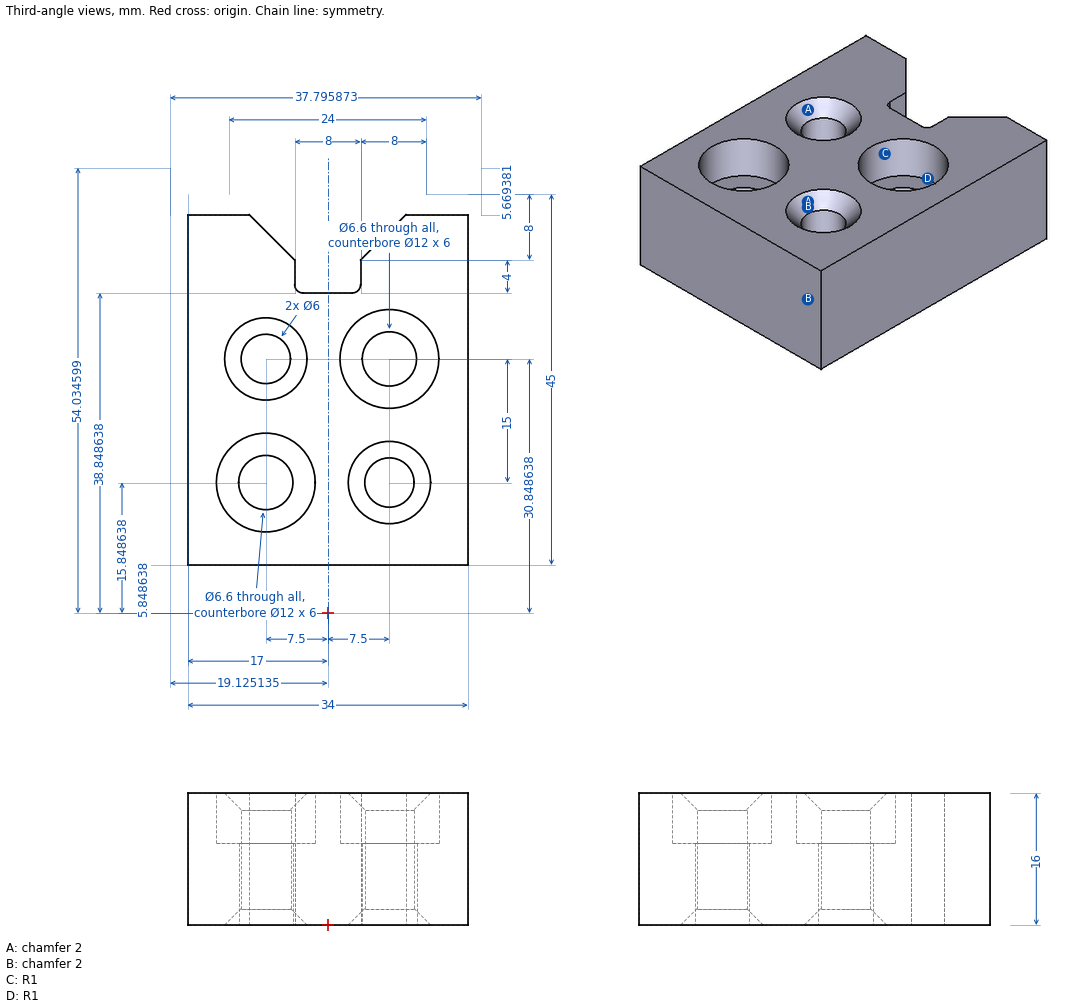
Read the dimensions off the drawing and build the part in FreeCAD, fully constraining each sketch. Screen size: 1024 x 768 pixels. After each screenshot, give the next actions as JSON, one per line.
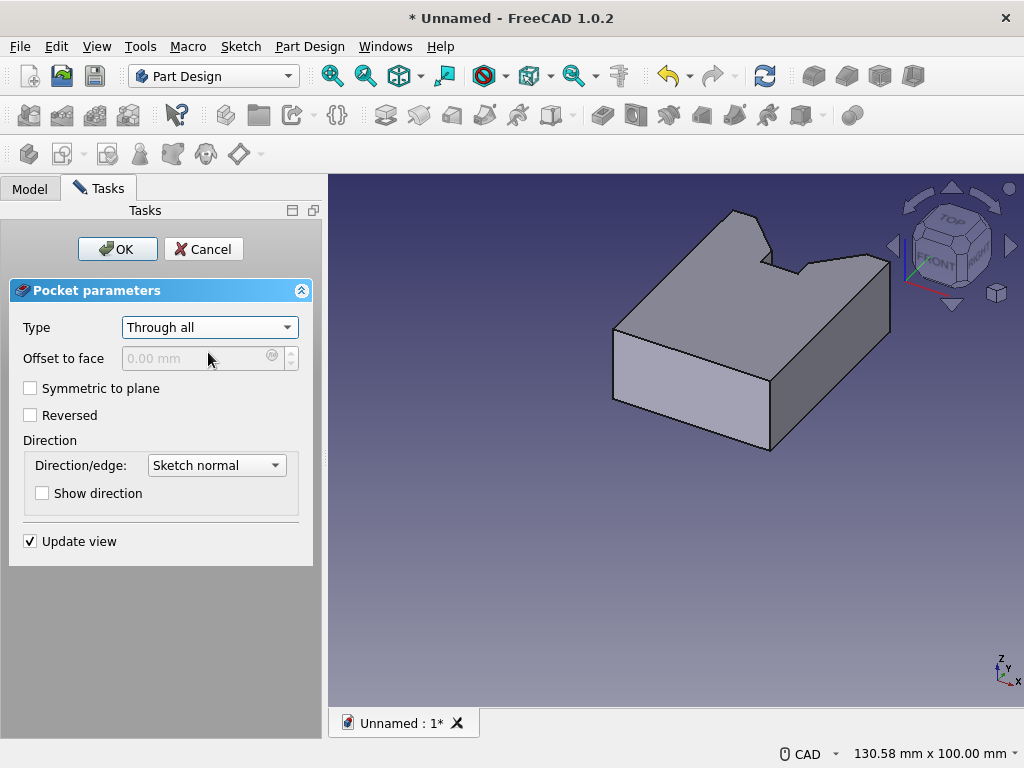
{"action": "left_click", "coordinate": [118, 249]}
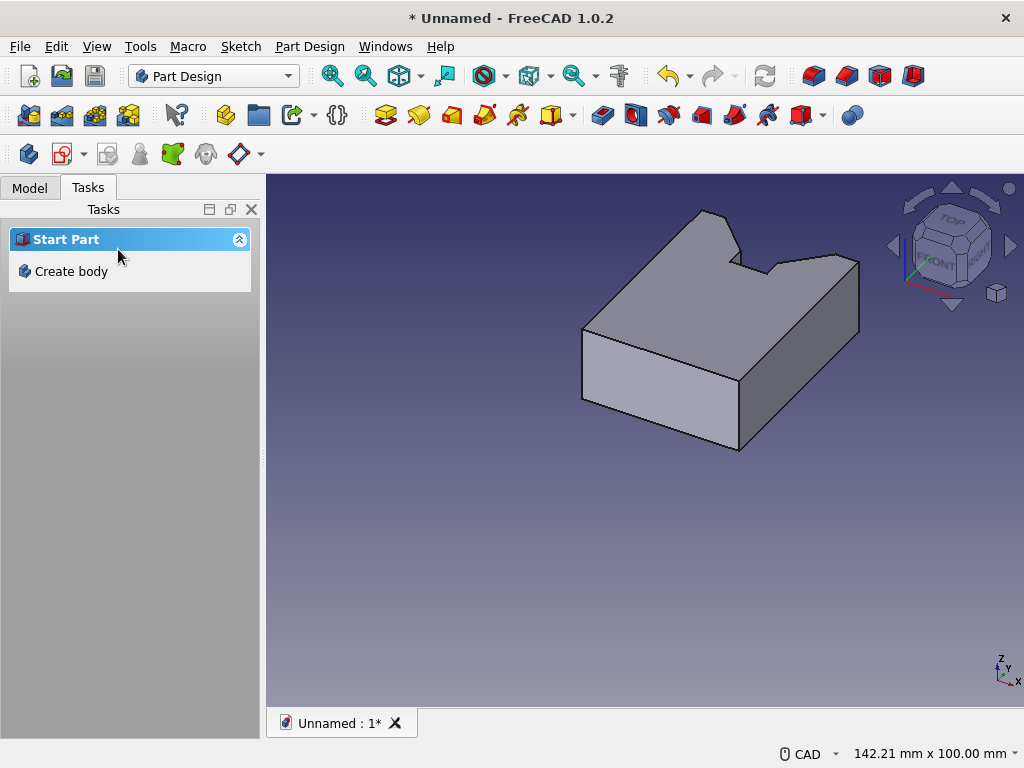
{"action": "left_click", "coordinate": [703, 312]}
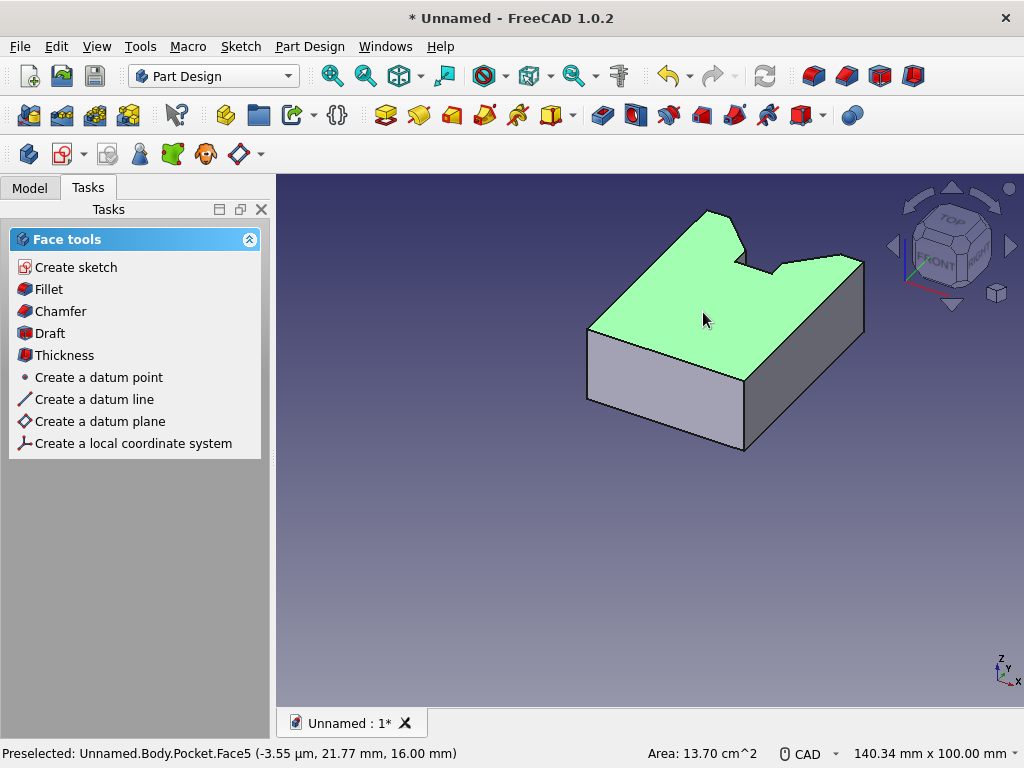
{"action": "left_click", "coordinate": [62, 154]}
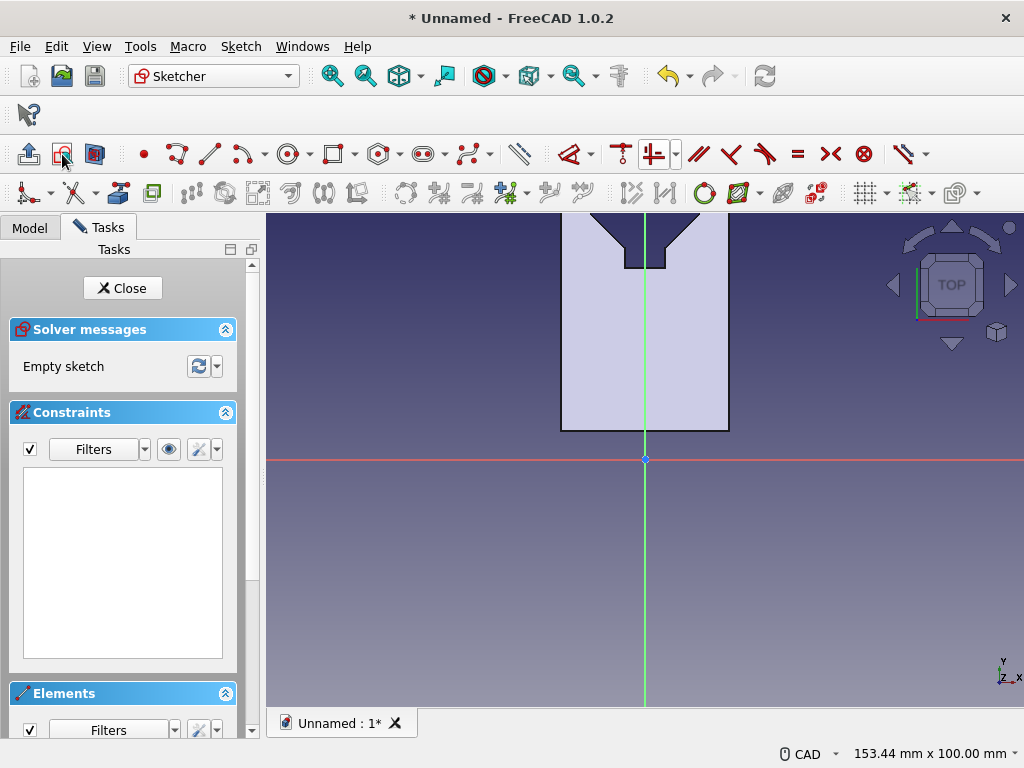
{"action": "scroll", "coordinate": [695, 289], "scroll_direction": "up", "scroll_amount": 11}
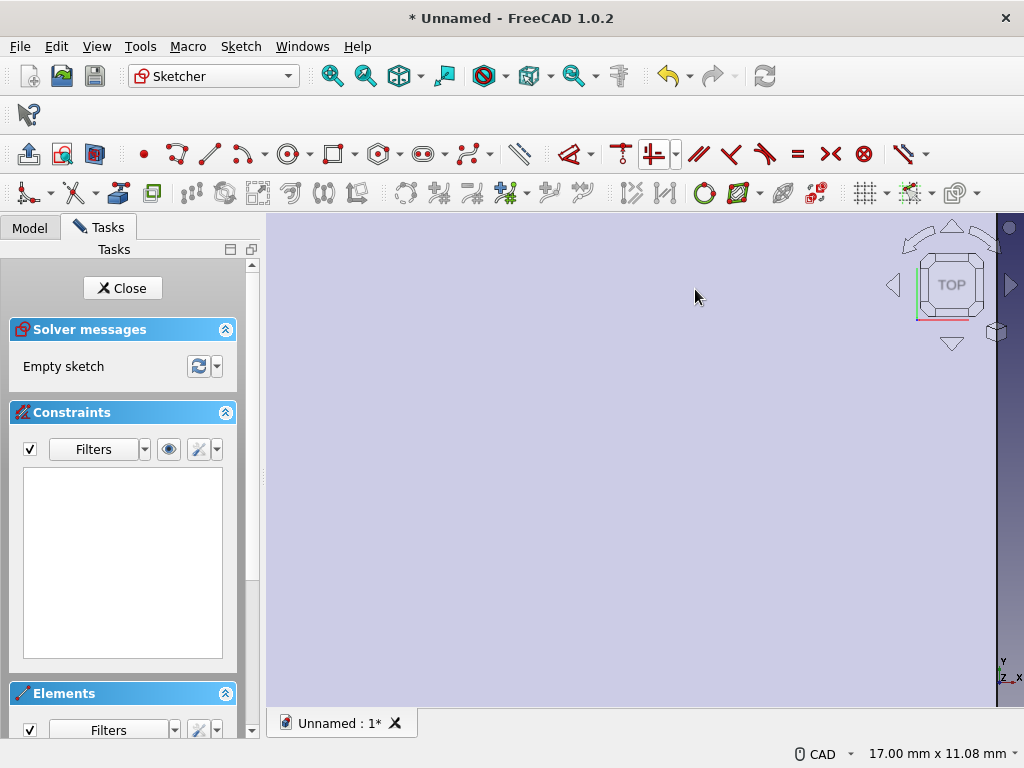
{"action": "left_click", "coordinate": [288, 154]}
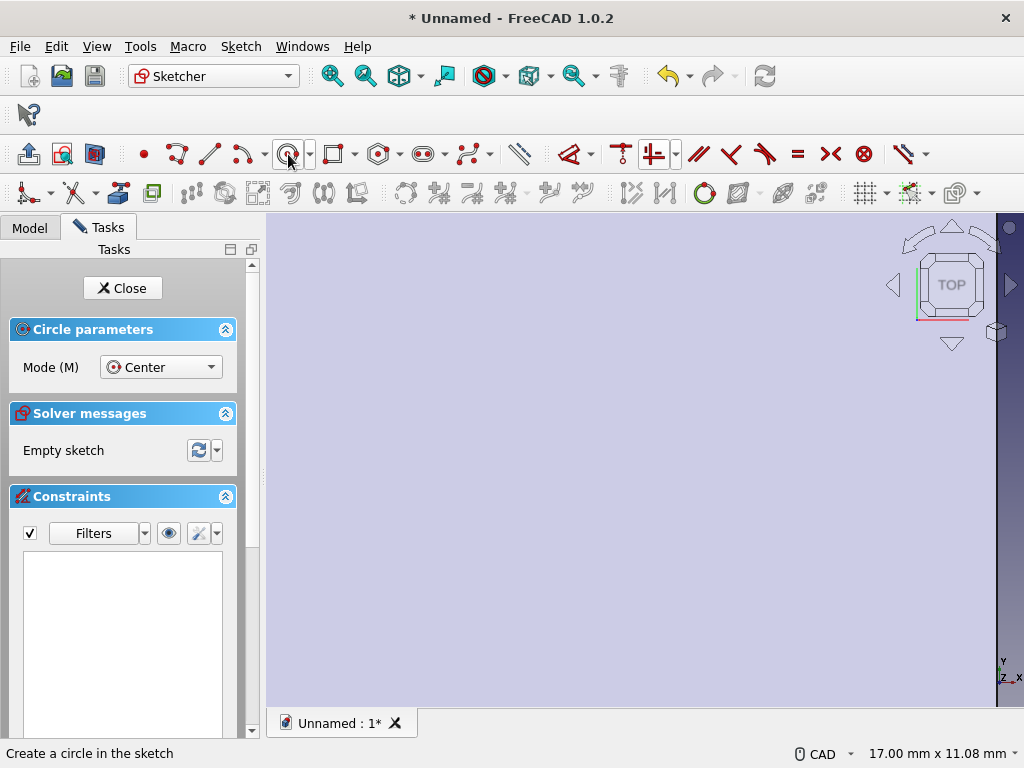
{"action": "left_click", "coordinate": [574, 456]}
{"action": "mouse_move", "coordinate": [678, 352]}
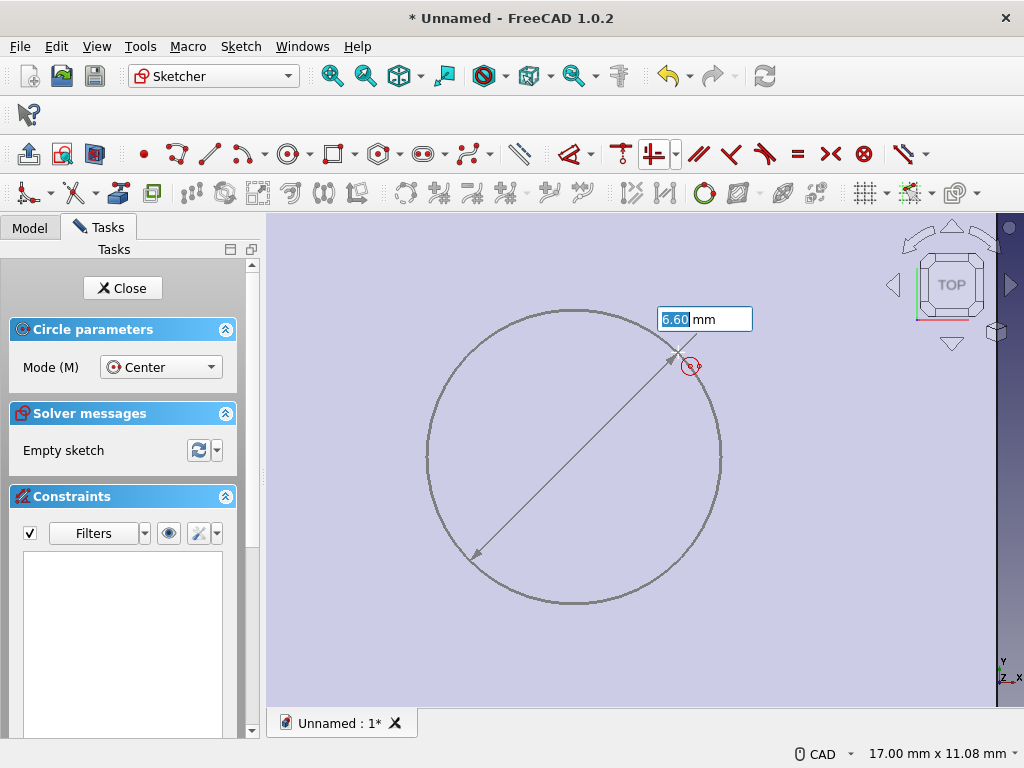
{"action": "type", "text": "6.6"}
{"action": "key", "text": "Return"}
{"action": "key", "text": "Escape"}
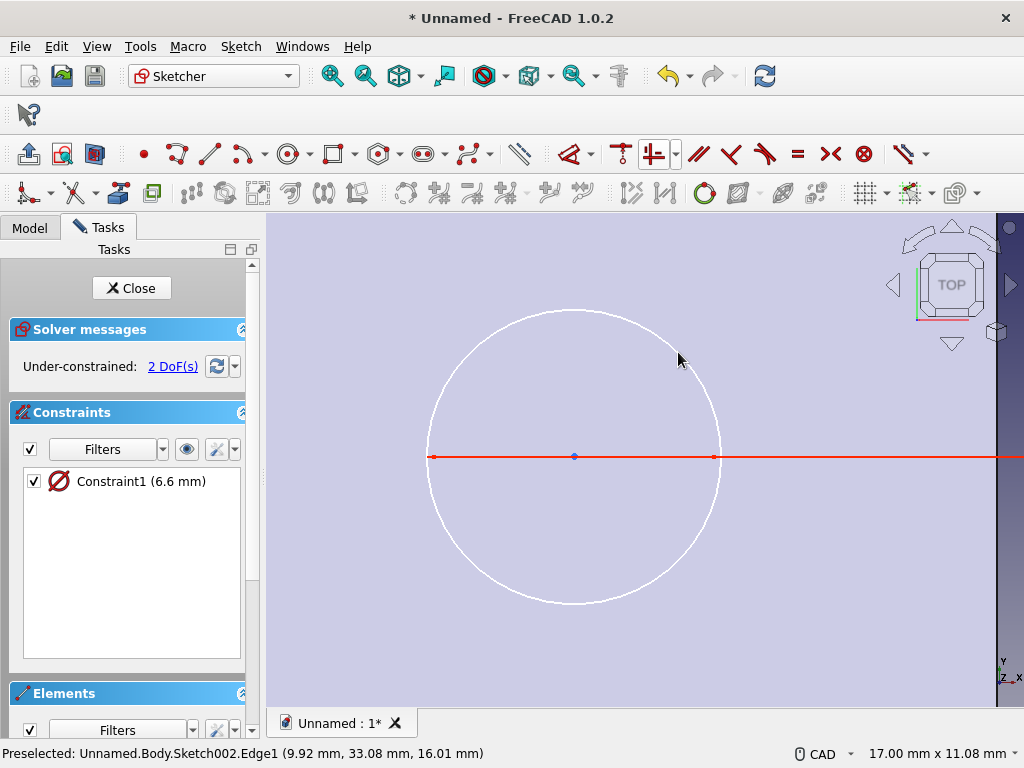
{"action": "key", "text": "d"}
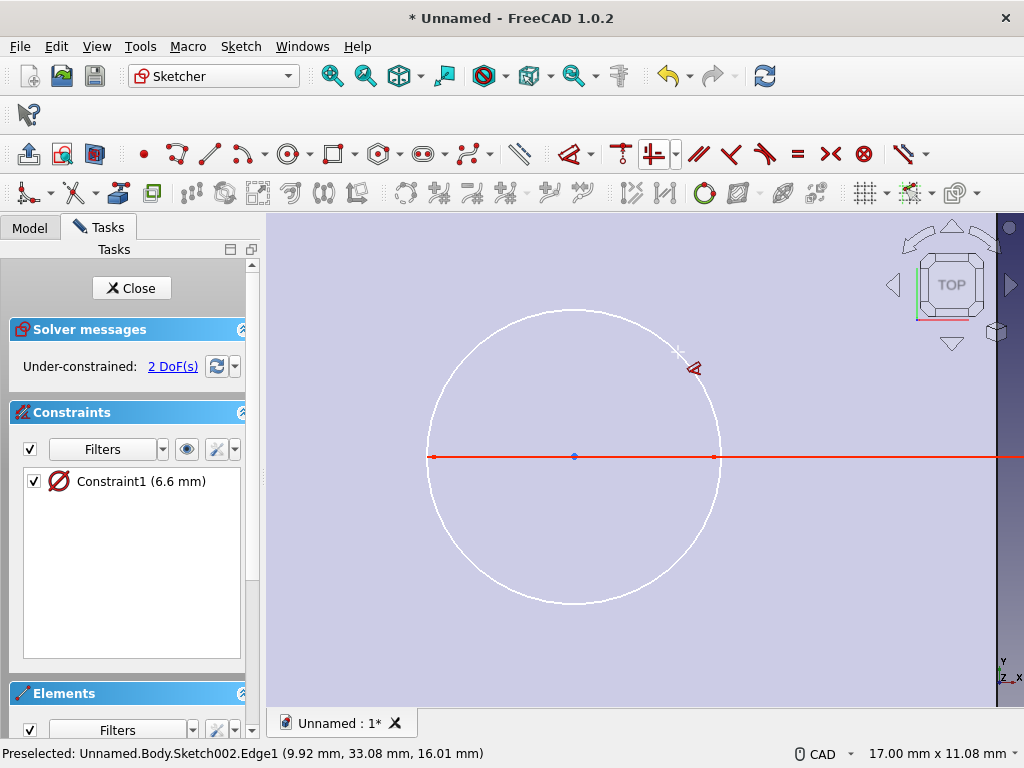
{"action": "left_click", "coordinate": [574, 457]}
{"action": "left_click", "coordinate": [370, 423]}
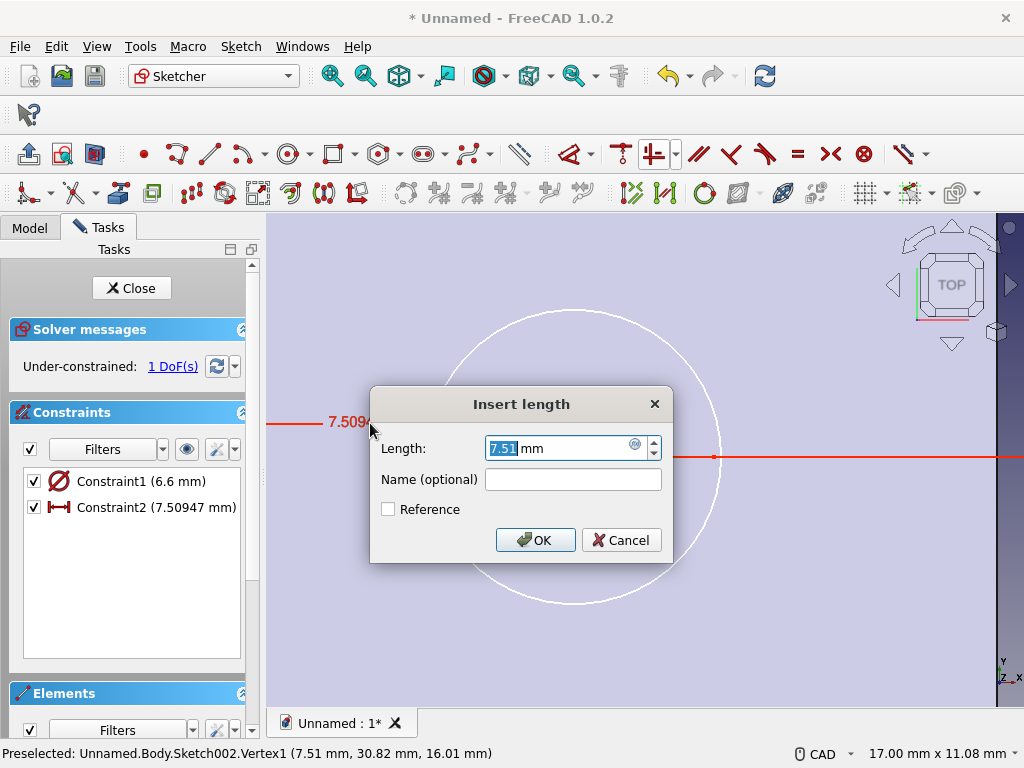
{"action": "type", "text": "7.5"}
{"action": "key", "text": "Return"}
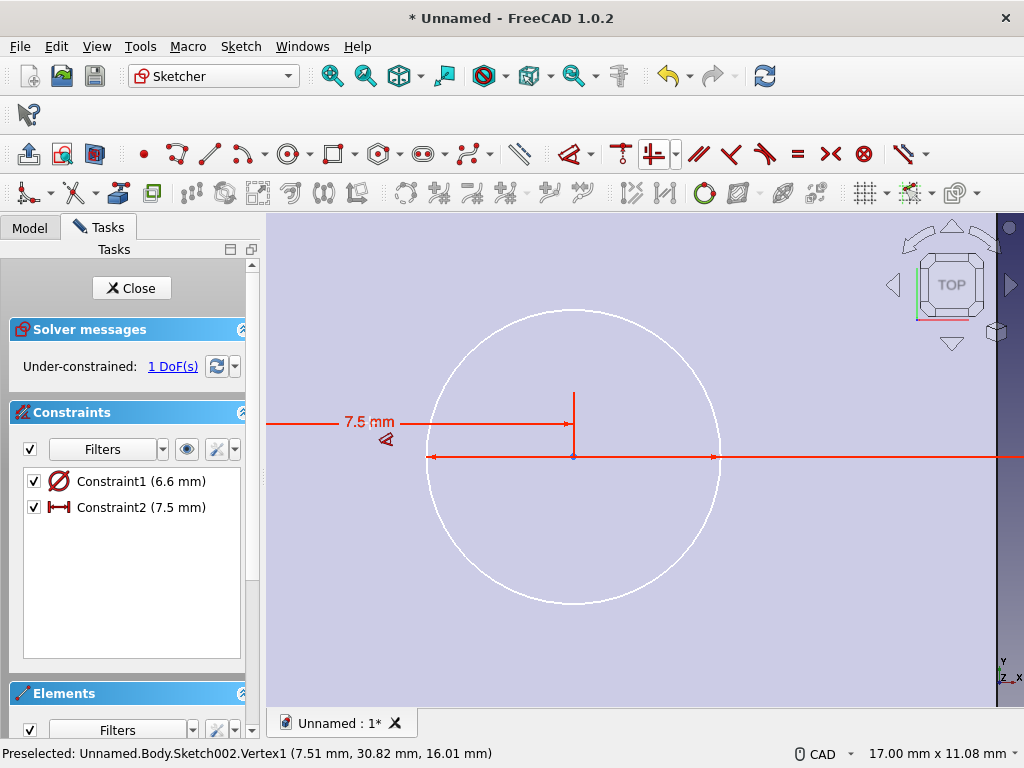
{"action": "left_click", "coordinate": [574, 457]}
{"action": "left_click", "coordinate": [608, 568]}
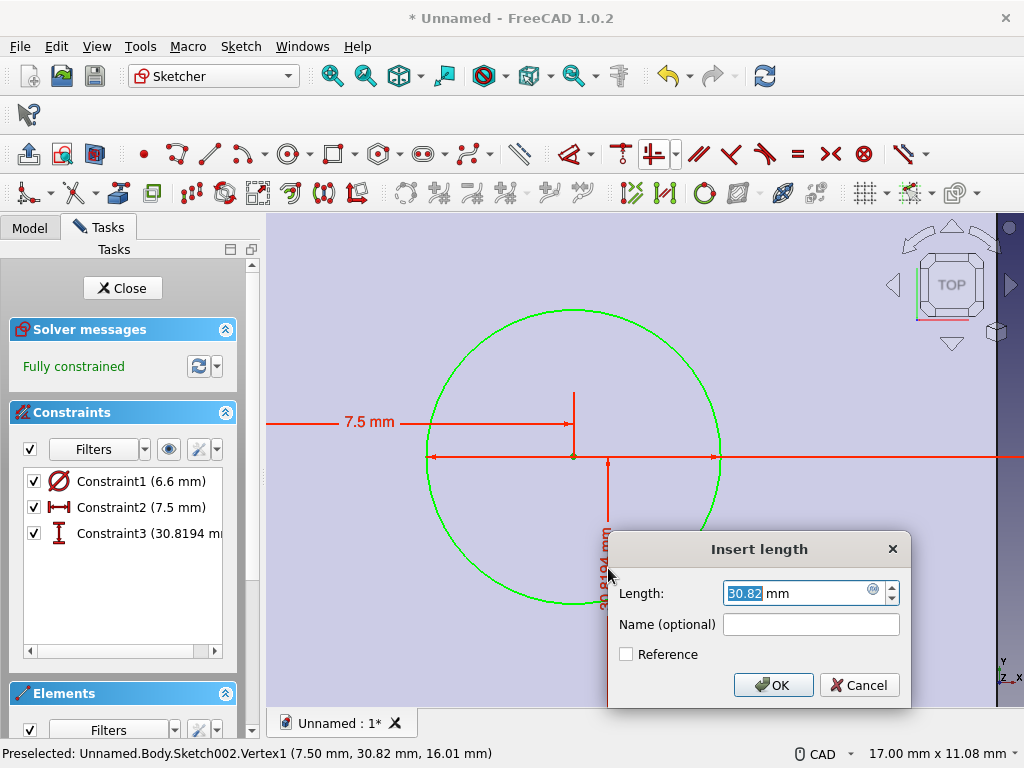
{"action": "type", "text": "30.848638"}
{"action": "key", "text": "Return"}
{"action": "key", "text": "Escape"}